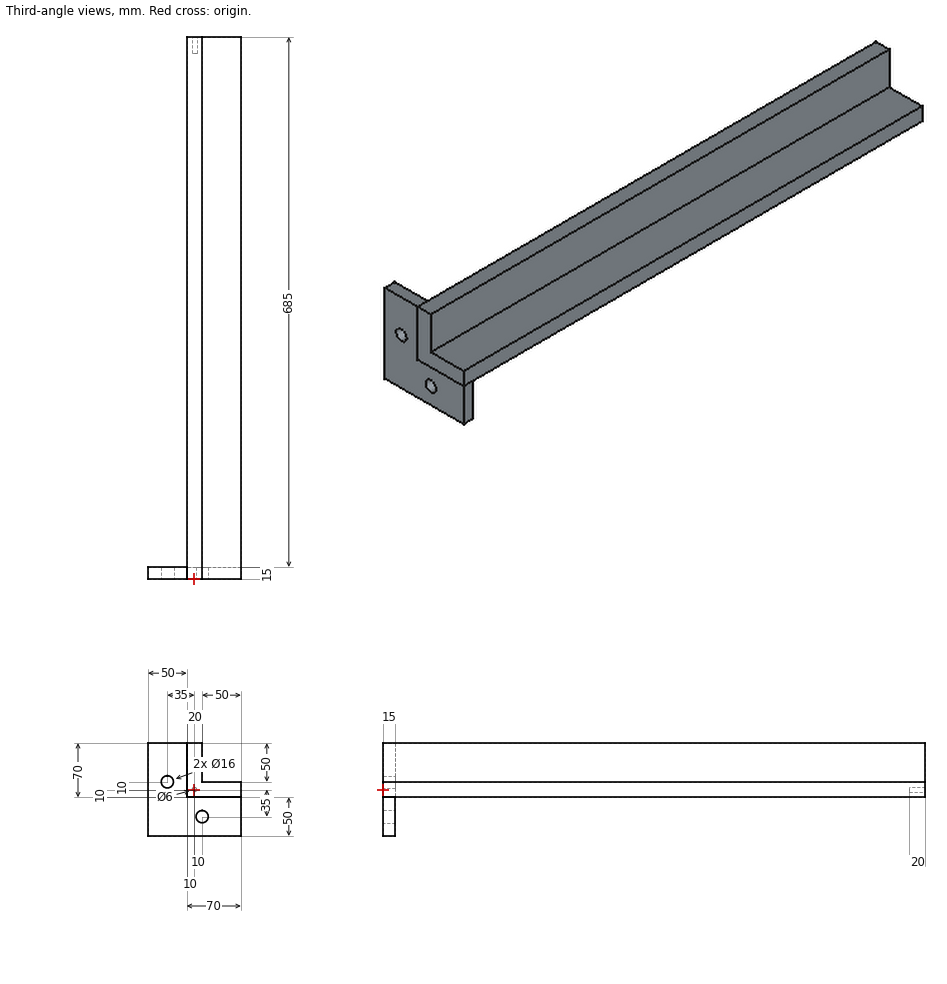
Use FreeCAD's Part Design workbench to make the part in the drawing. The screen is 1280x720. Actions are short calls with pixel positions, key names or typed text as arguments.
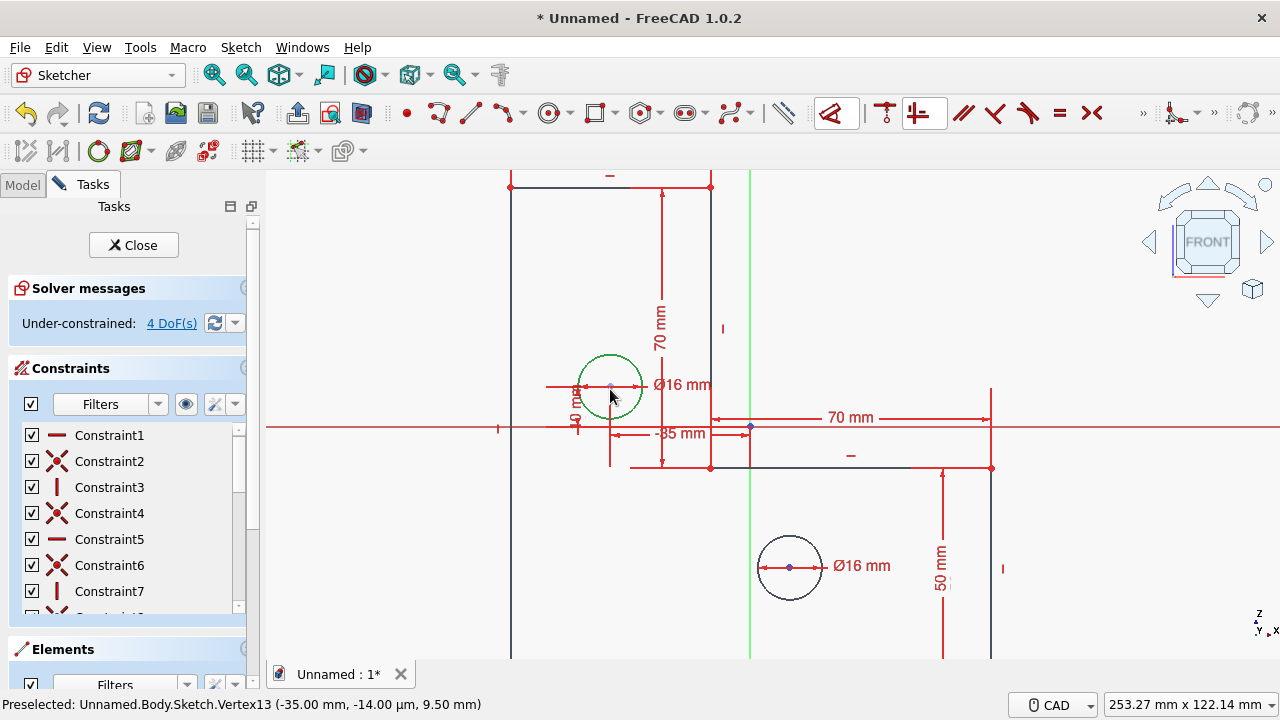
click(790, 568)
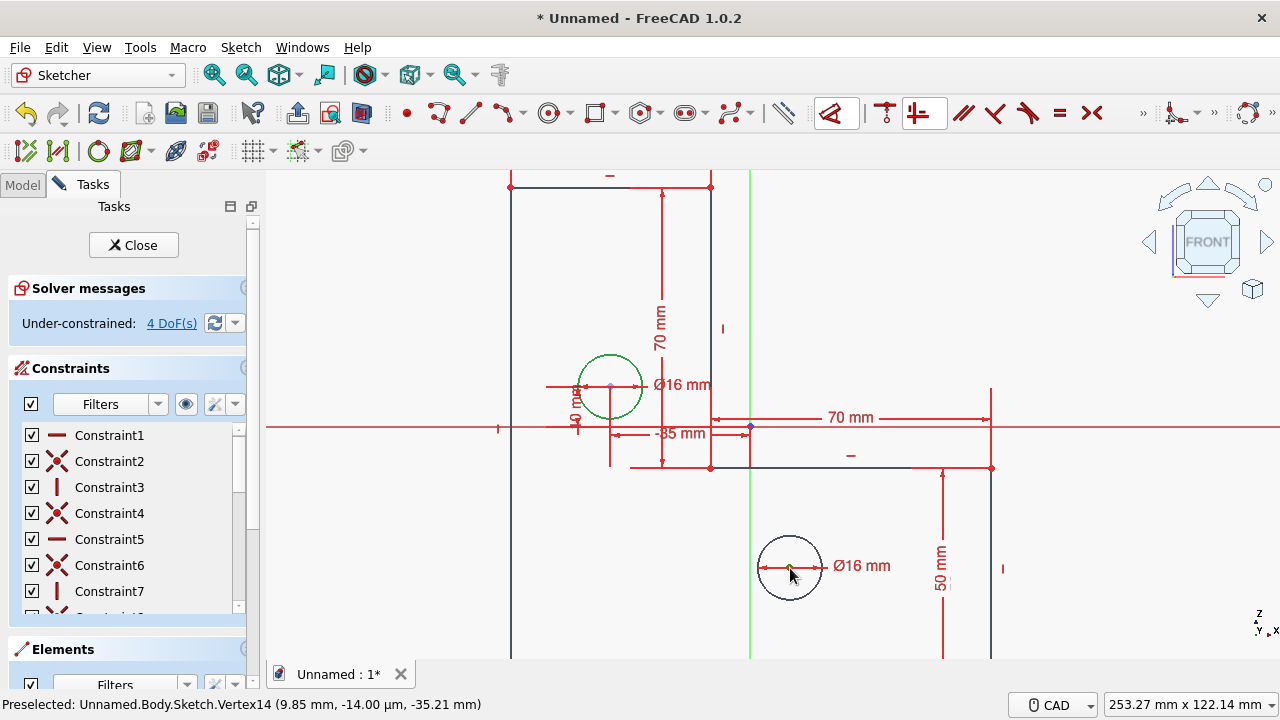
key(l)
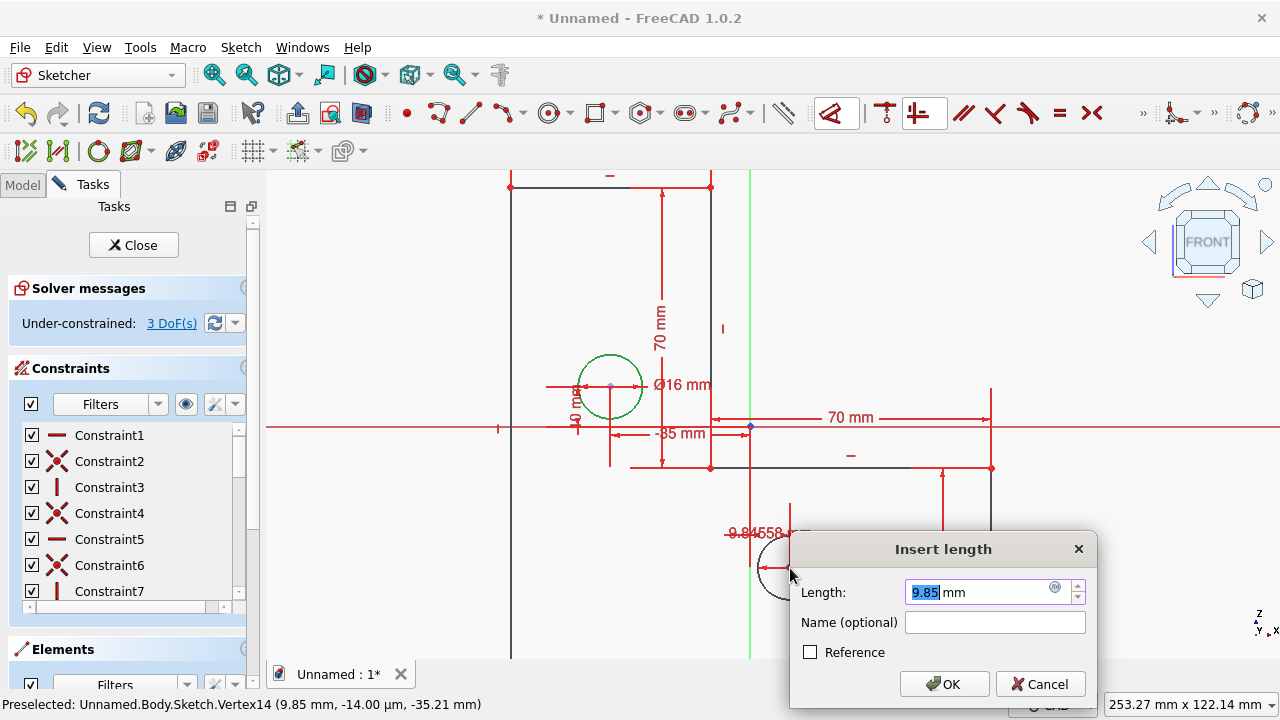
text(10)
key(Return)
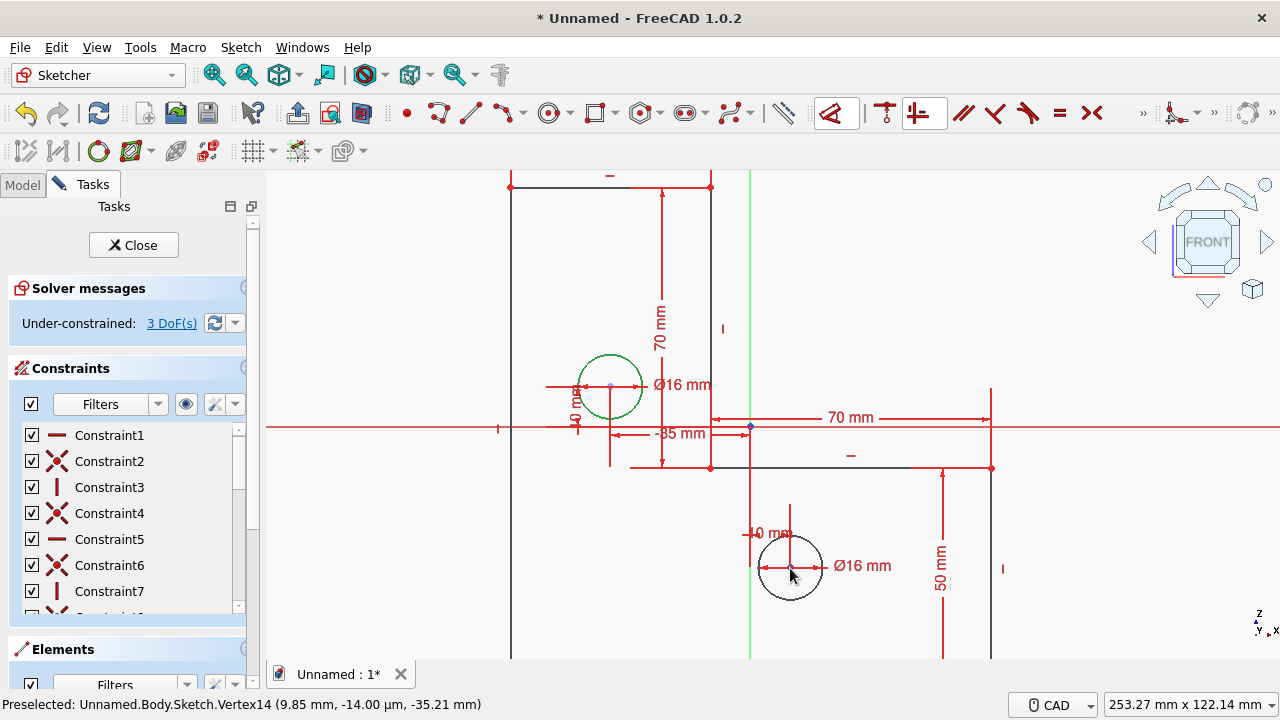
click(790, 568)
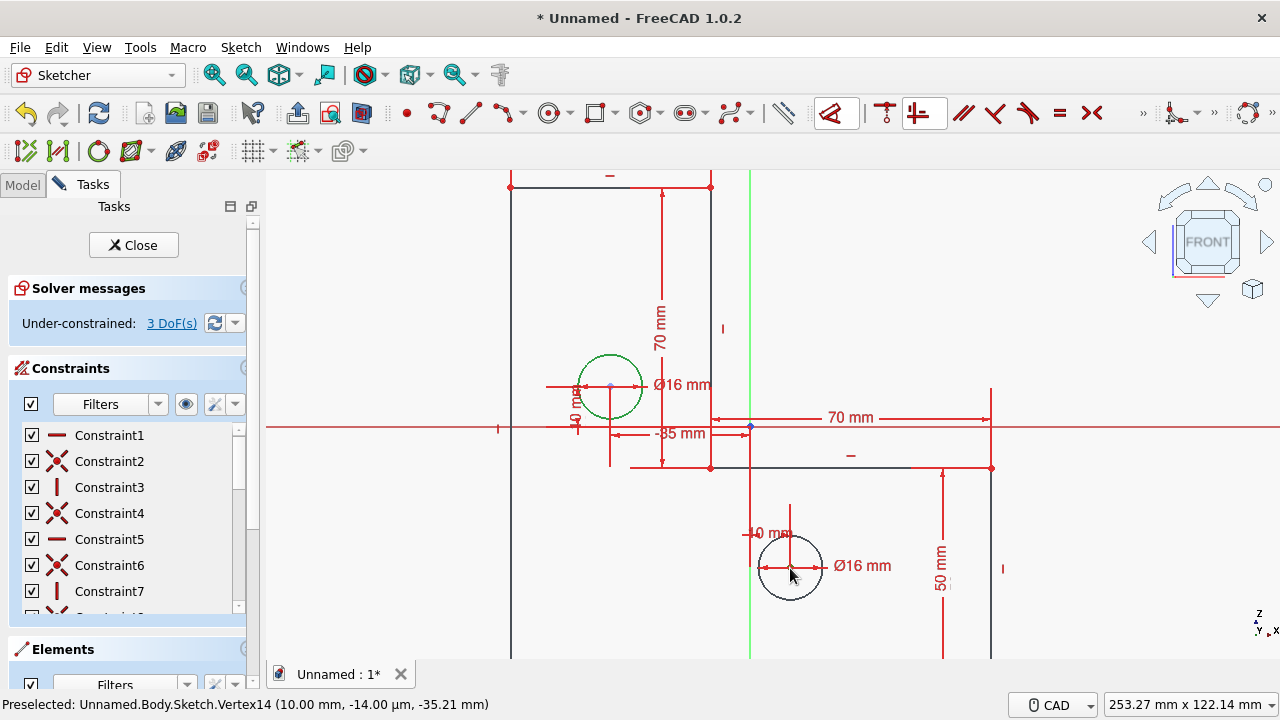
click(854, 114)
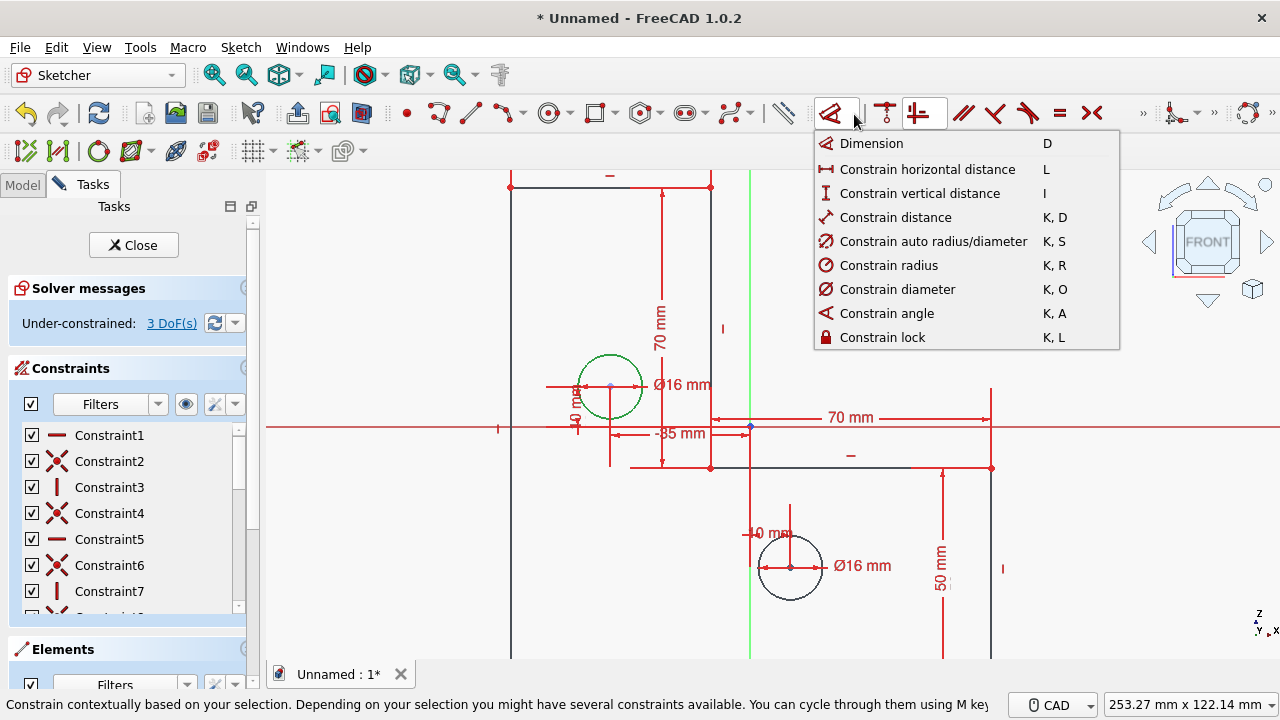
click(967, 193)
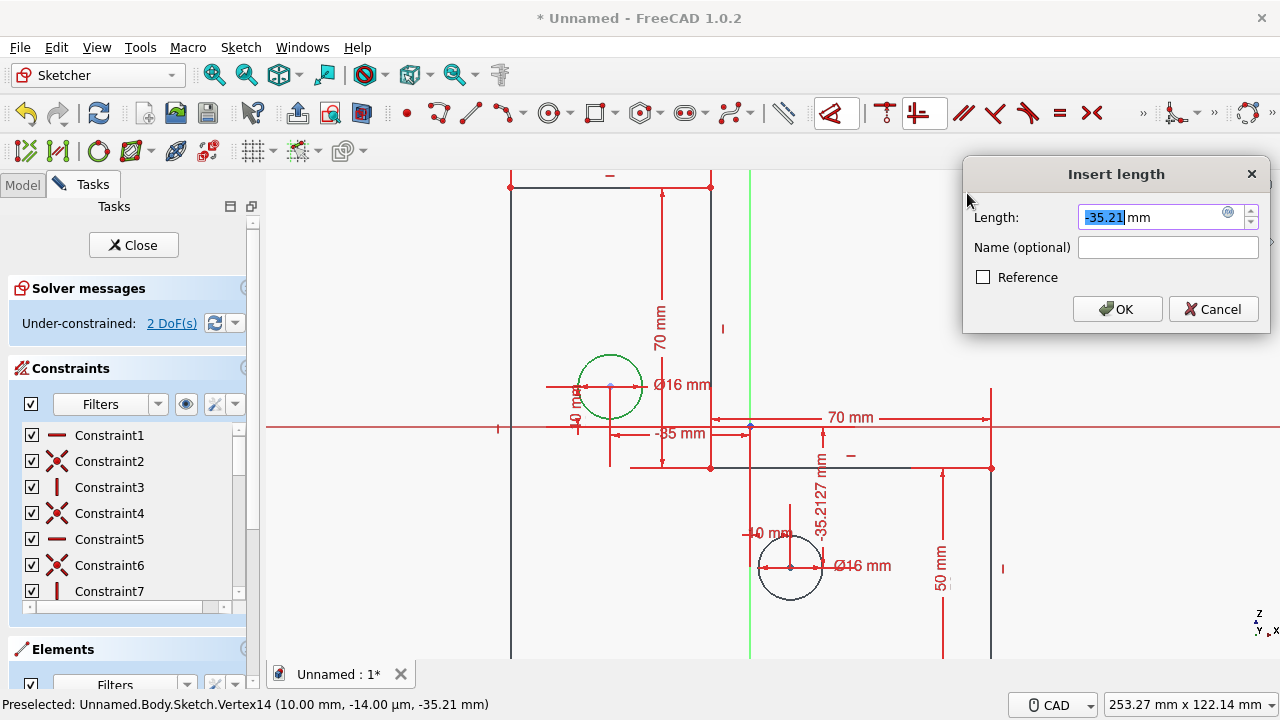
text(-35)
key(Return)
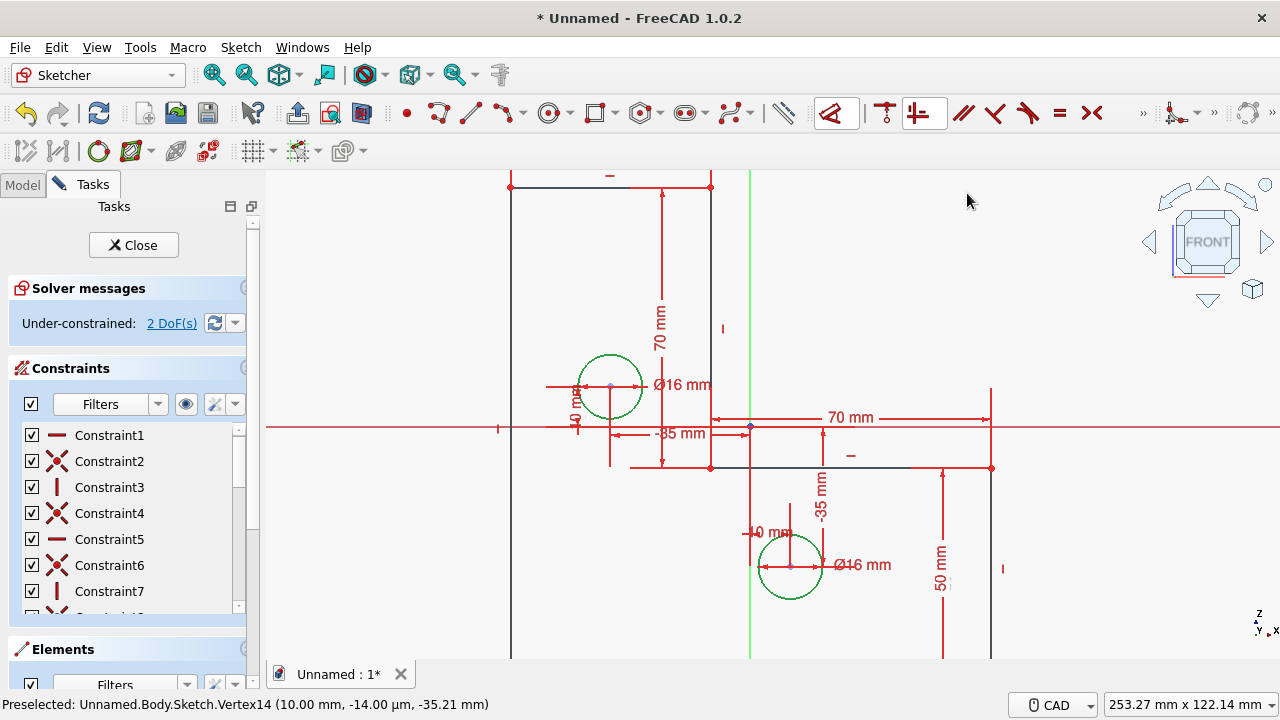
click(711, 468)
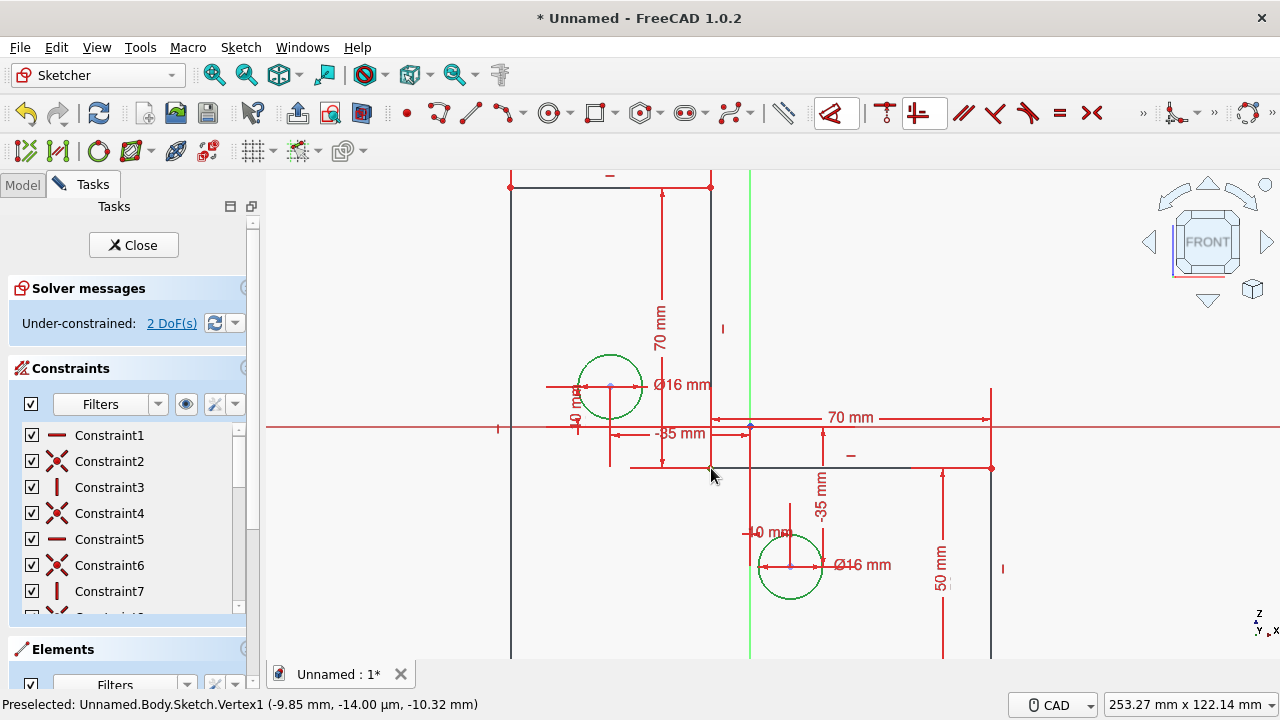
key(l)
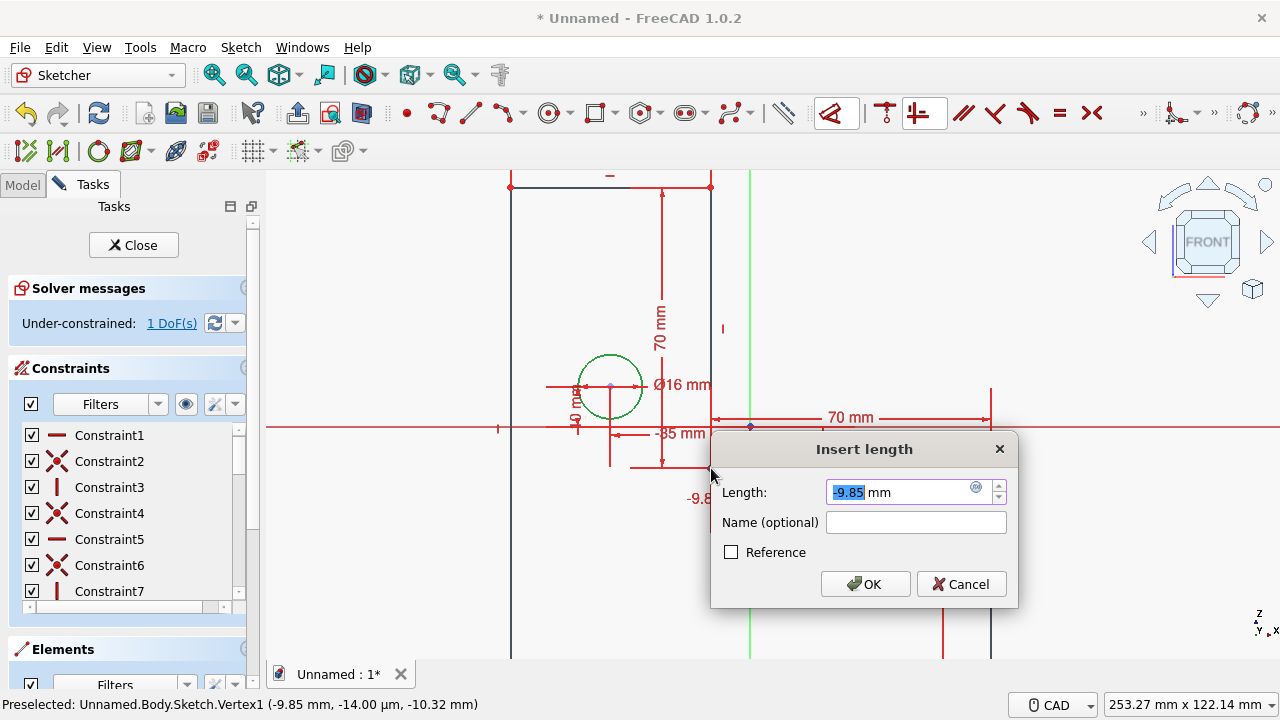
text(-10)
key(Return)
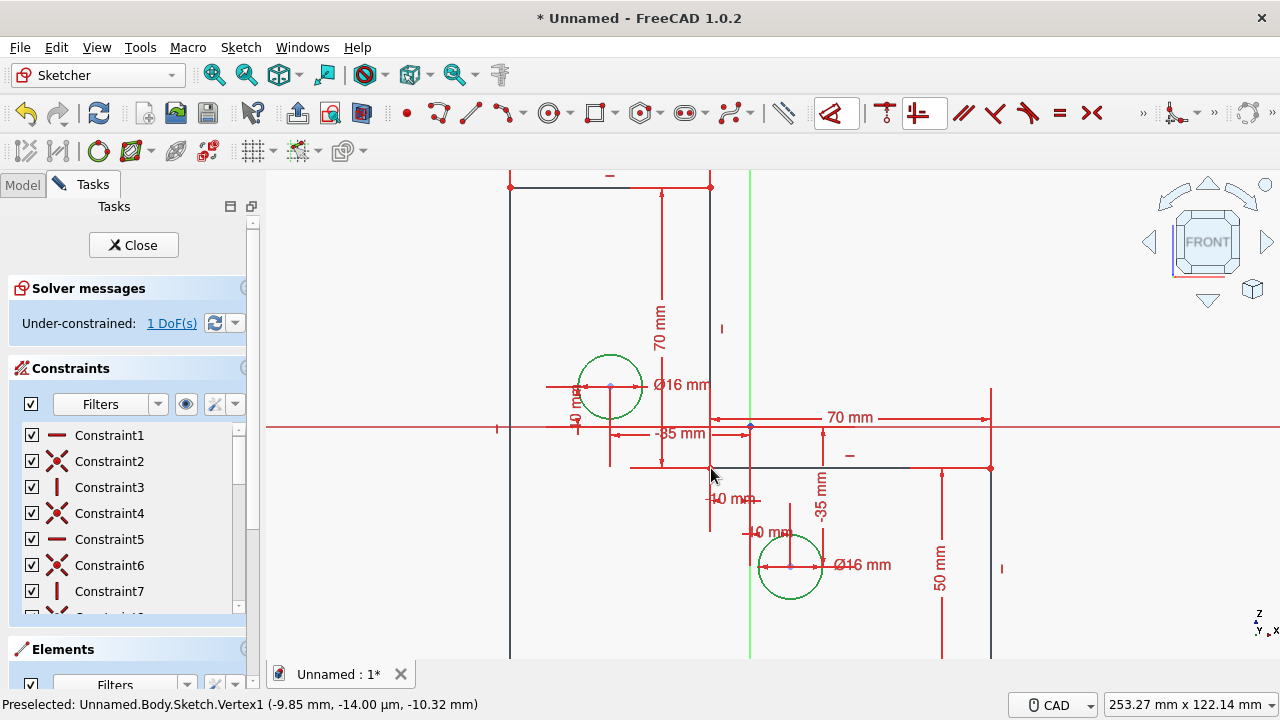
click(710, 468)